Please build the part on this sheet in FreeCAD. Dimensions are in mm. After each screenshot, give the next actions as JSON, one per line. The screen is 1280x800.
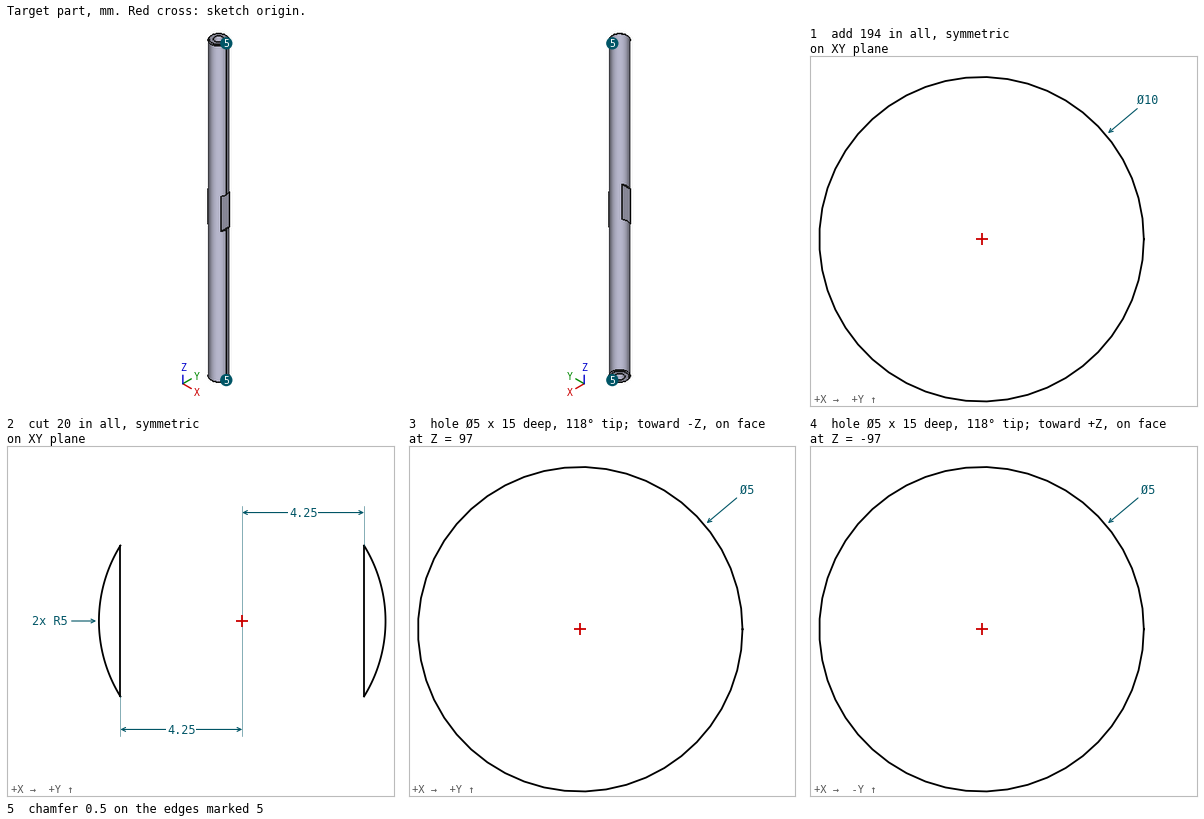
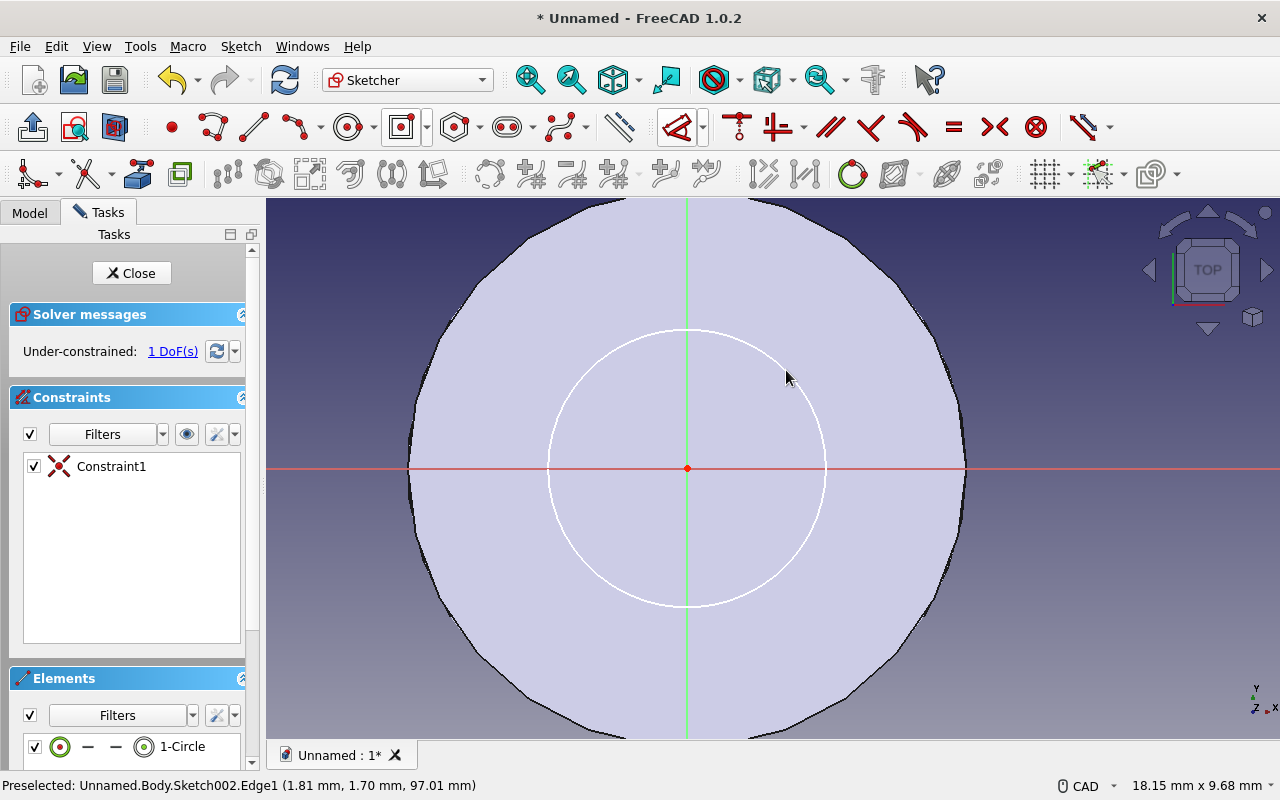
{"action": "left_click", "coordinate": [785, 370]}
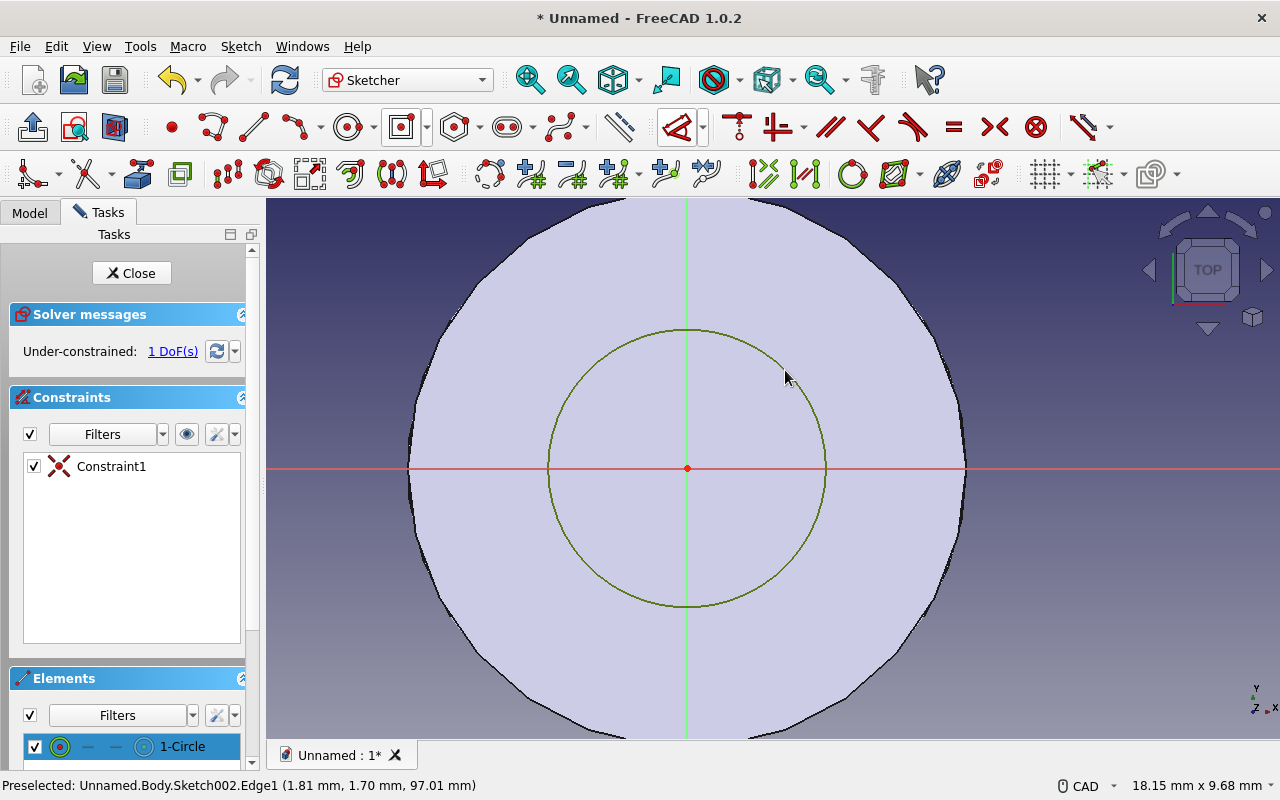
{"action": "key", "text": "k o"}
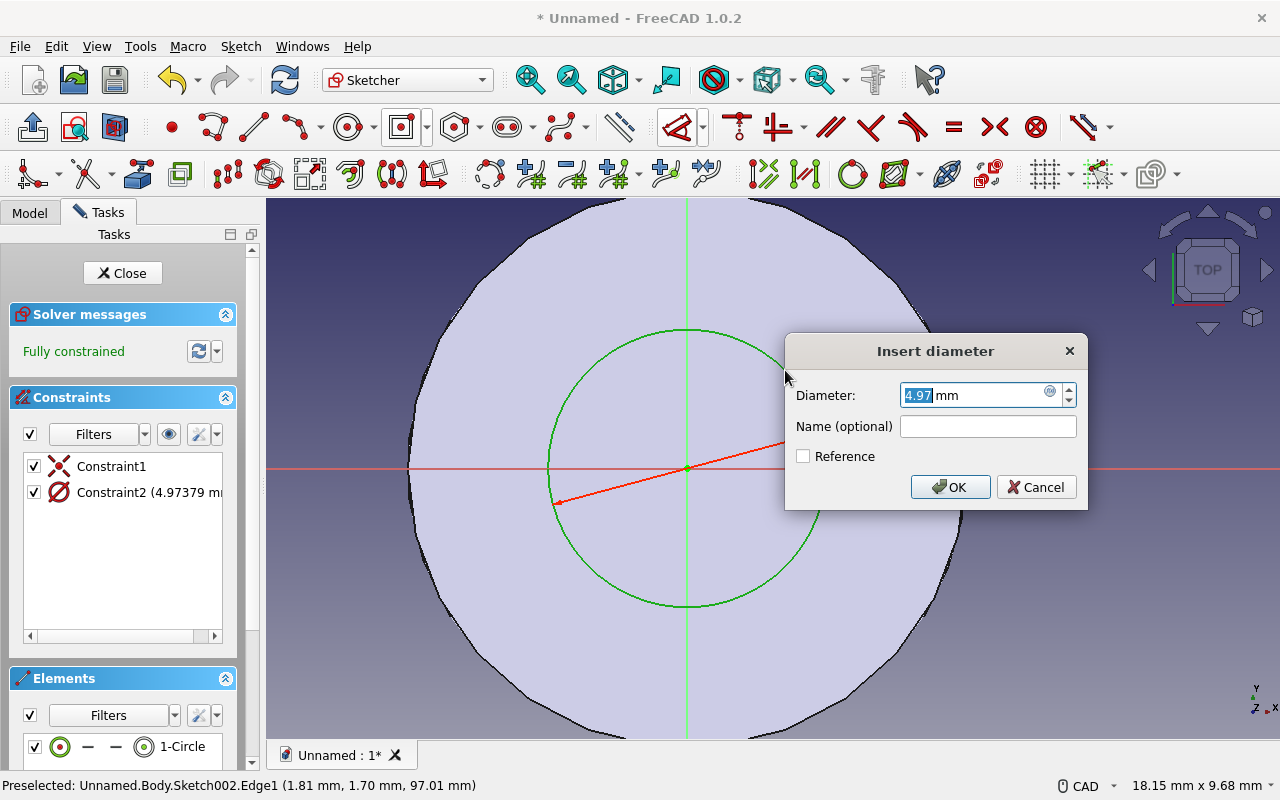
{"action": "type", "text": "5"}
{"action": "key", "text": "Return"}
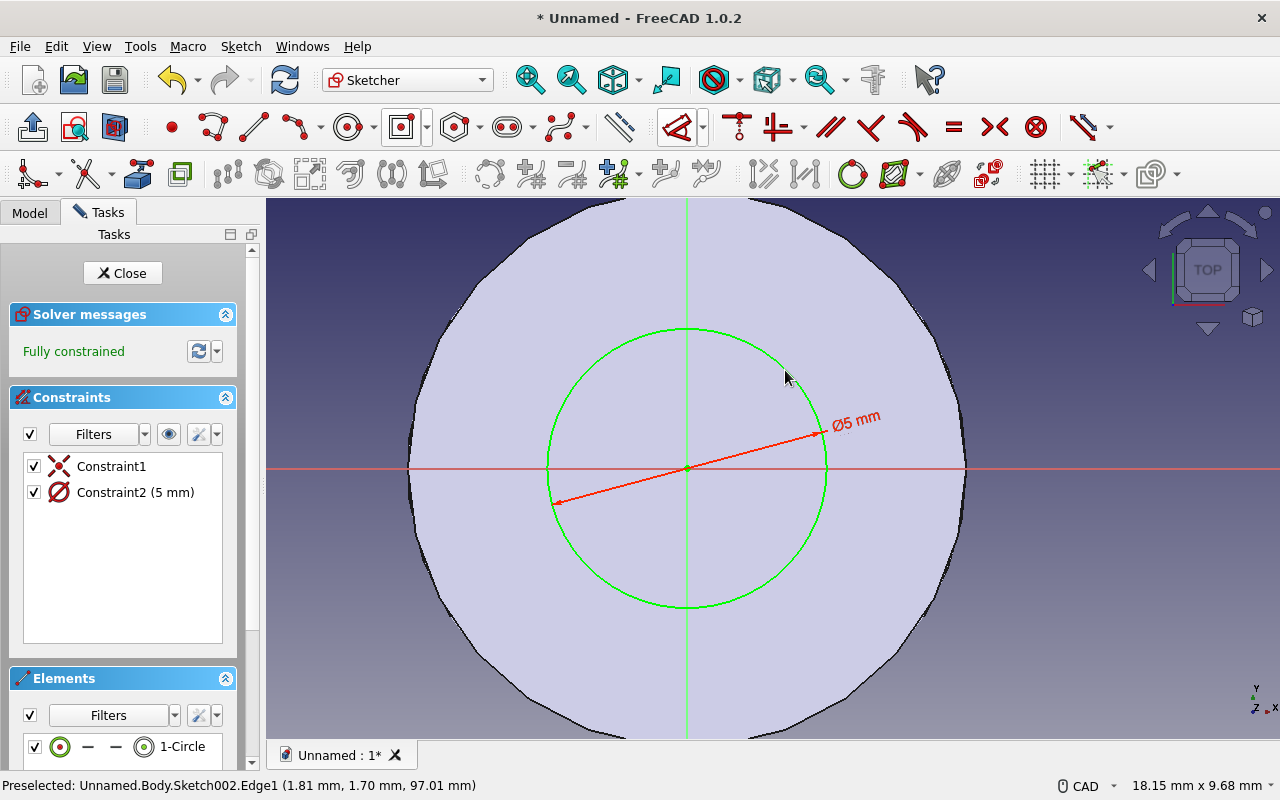
{"action": "left_click", "coordinate": [123, 273]}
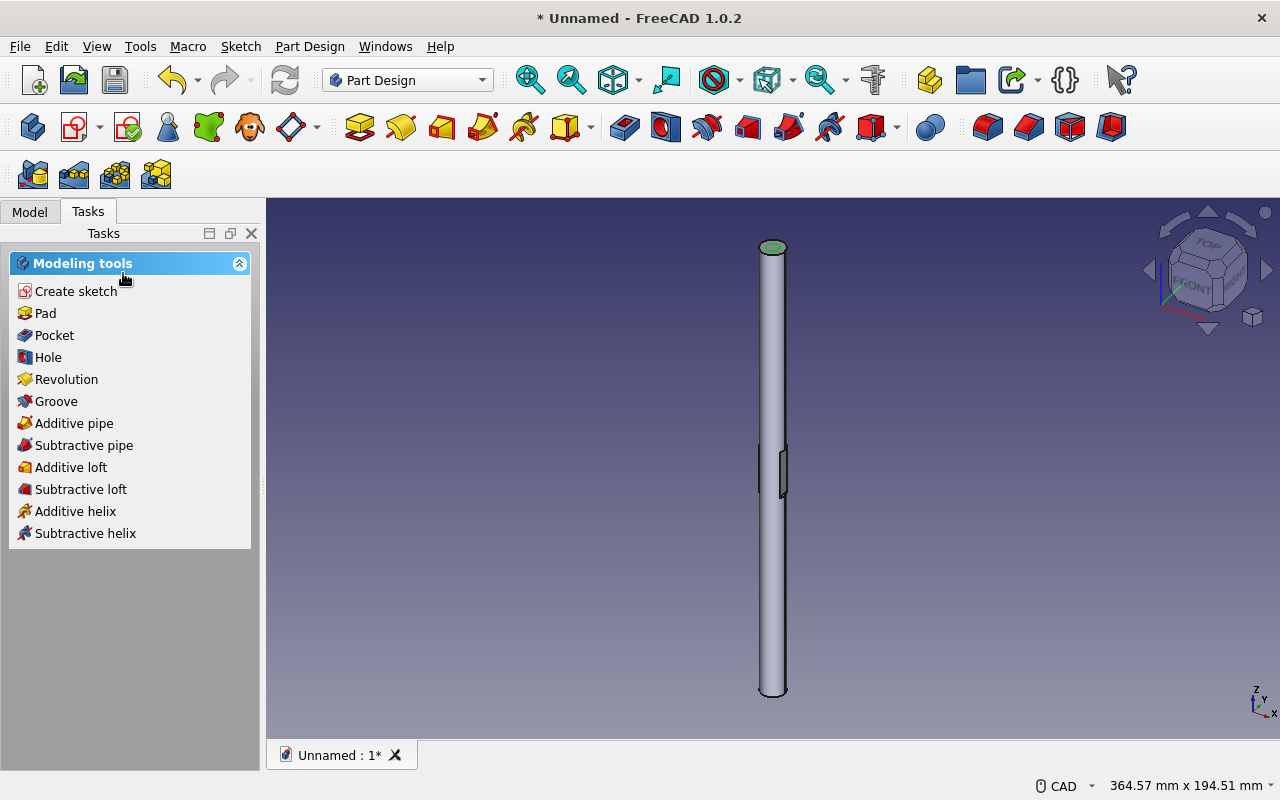
{"action": "left_click", "coordinate": [666, 128]}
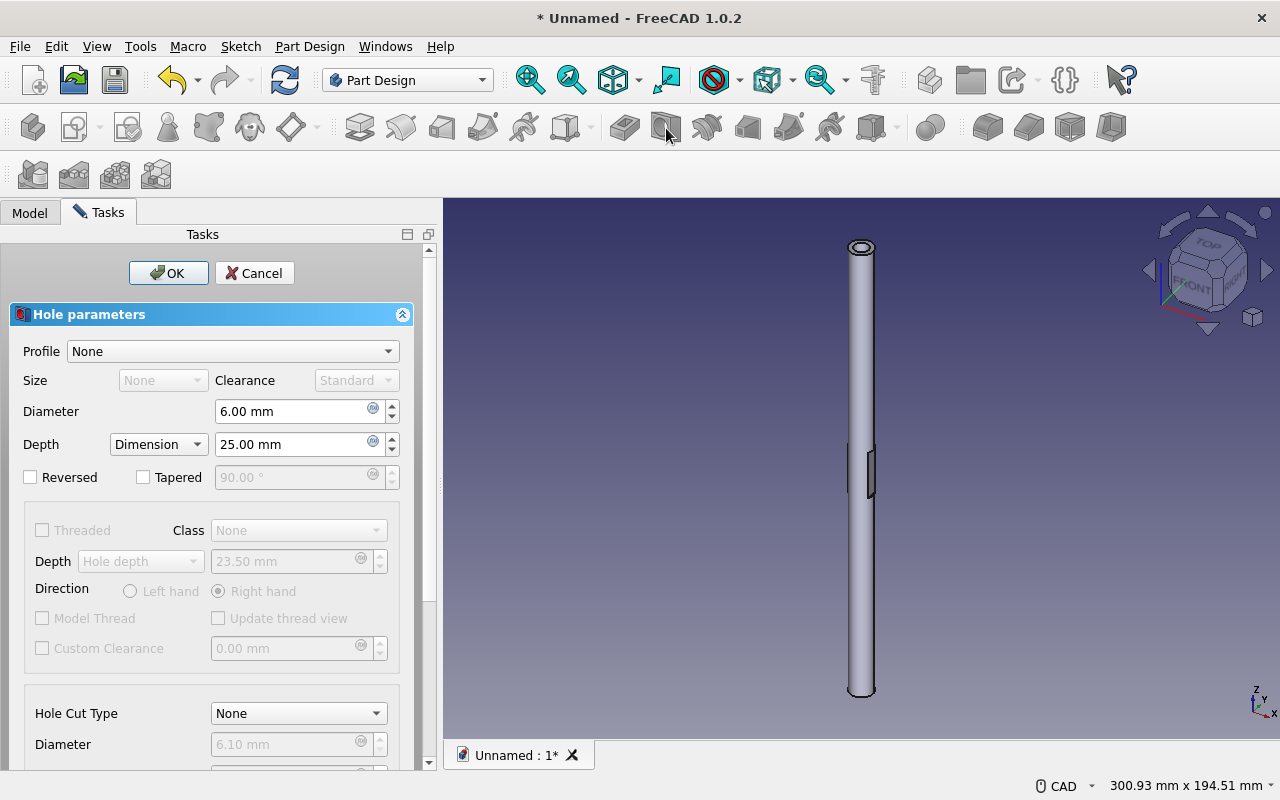
{"action": "triple_click", "coordinate": [300, 412]}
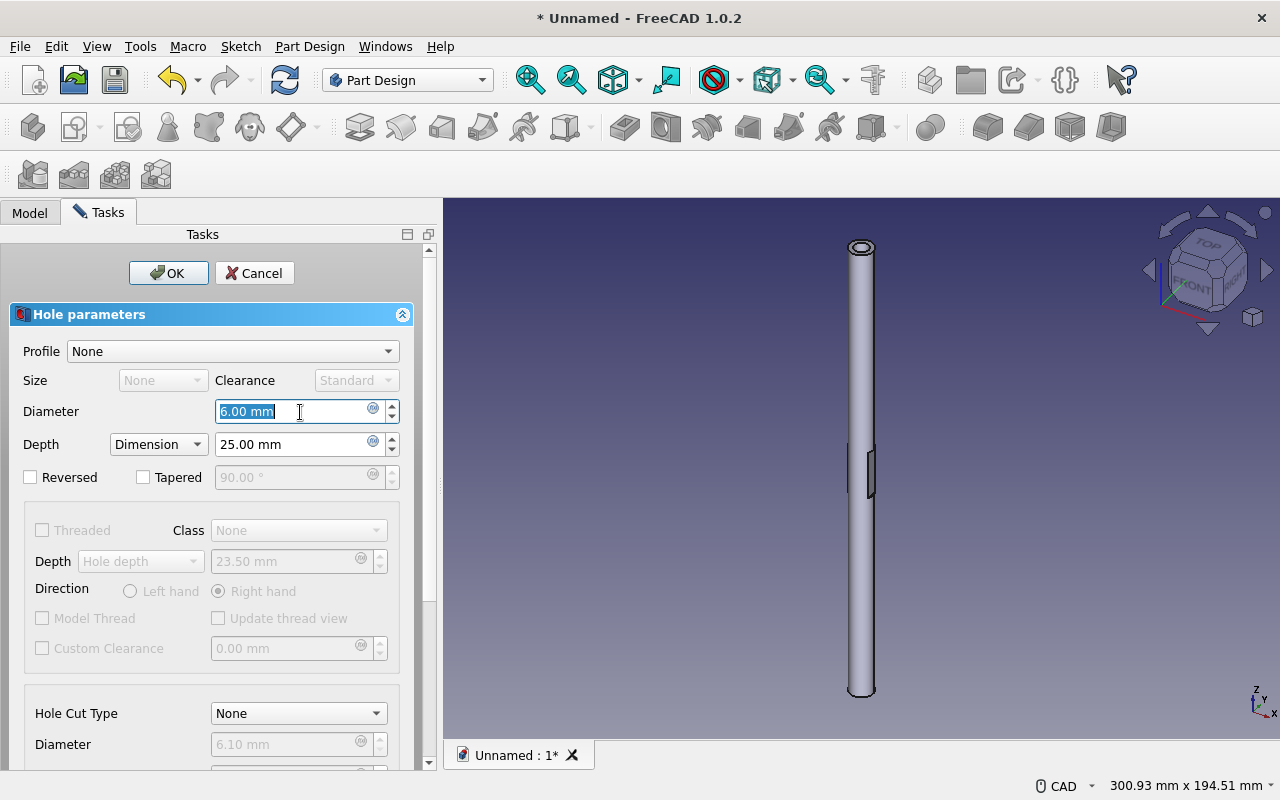
{"action": "type", "text": "5"}
{"action": "key", "text": "Tab"}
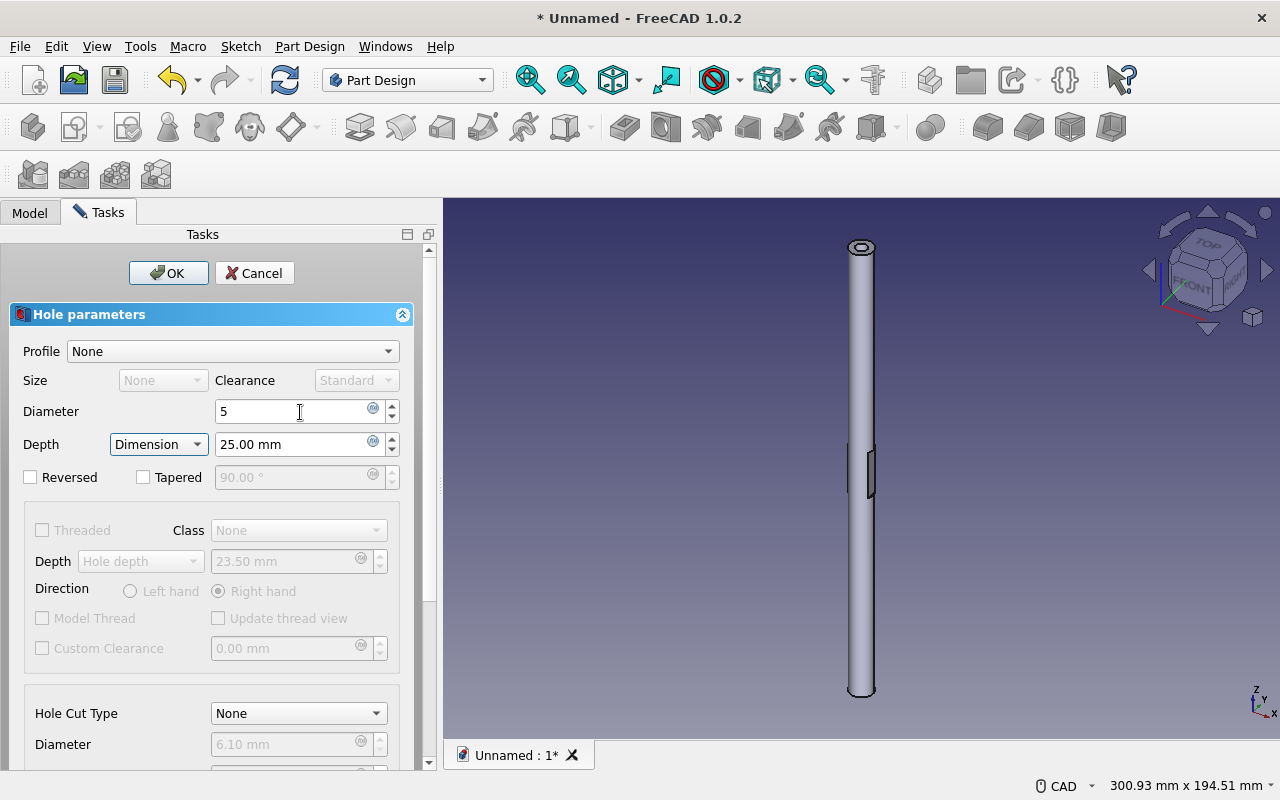
{"action": "triple_click", "coordinate": [300, 444]}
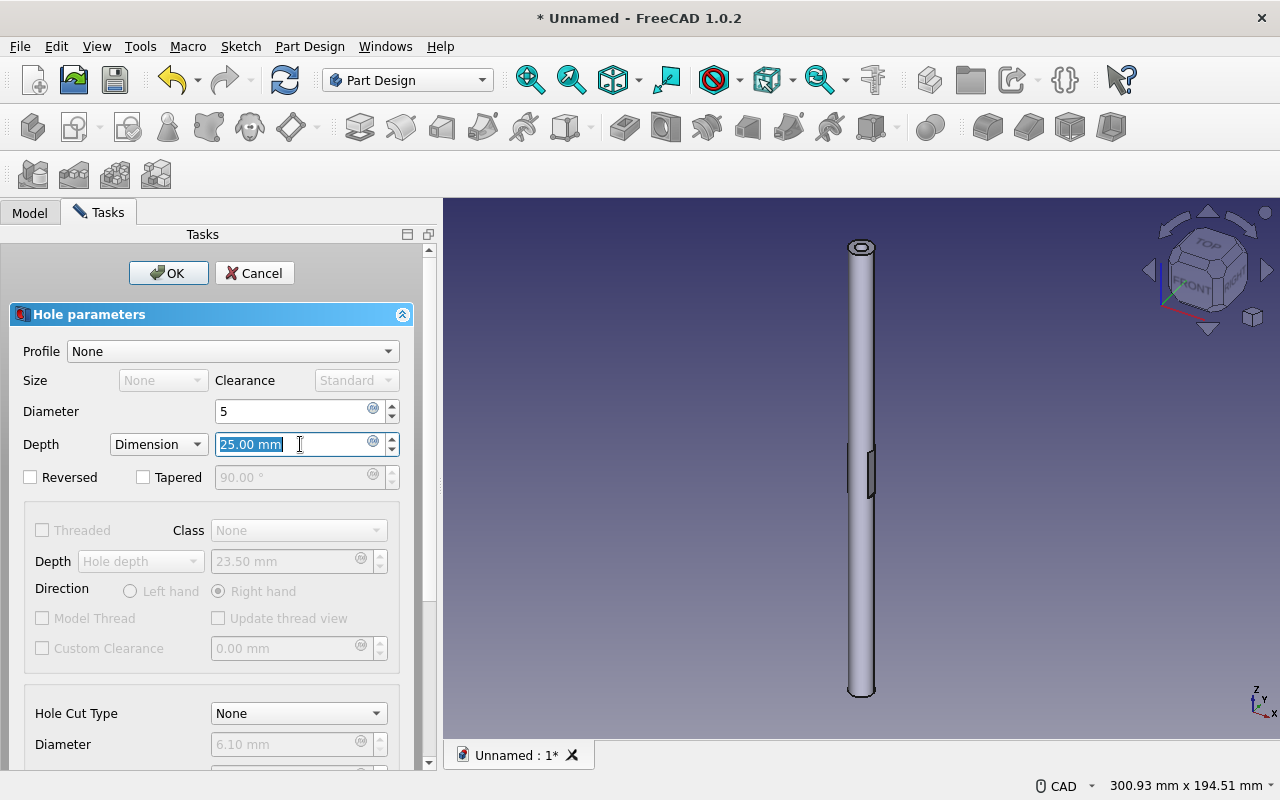
{"action": "type", "text": "15"}
{"action": "key", "text": "Tab"}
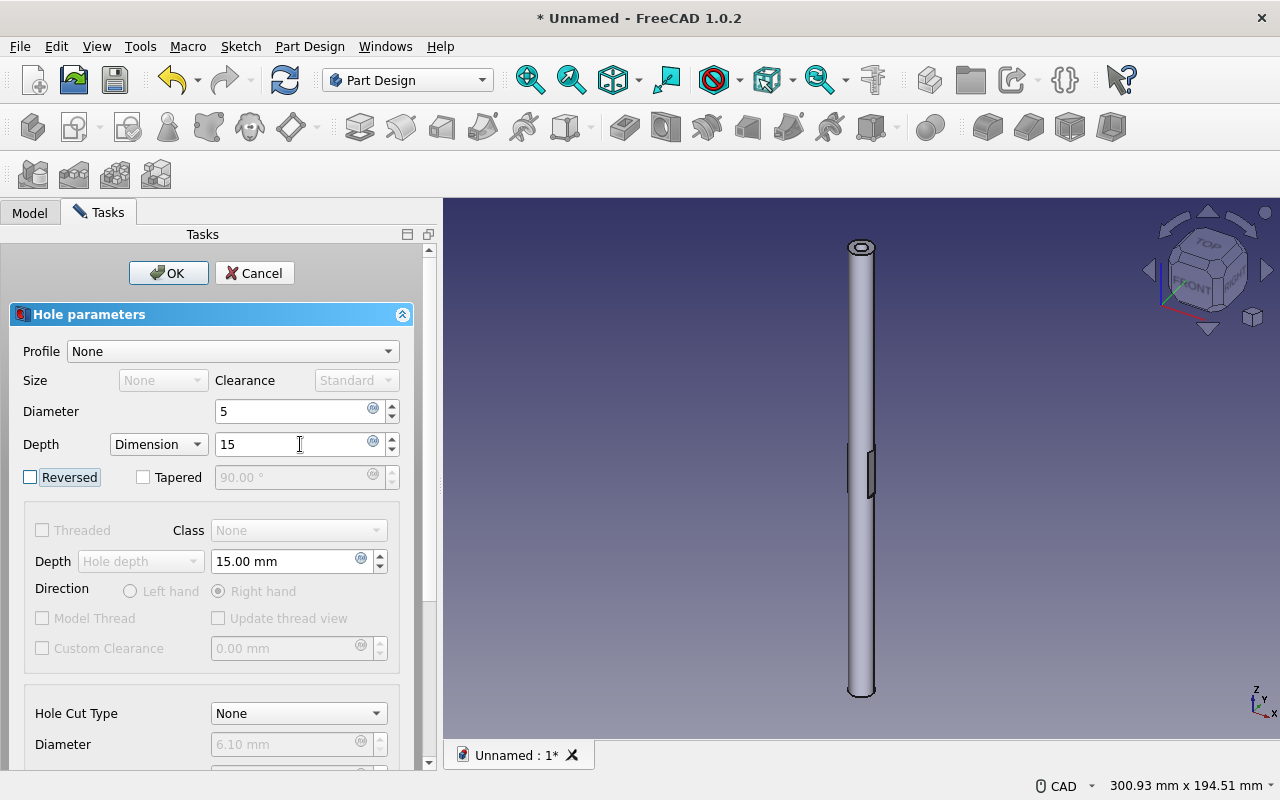
{"action": "left_click", "coordinate": [169, 273]}